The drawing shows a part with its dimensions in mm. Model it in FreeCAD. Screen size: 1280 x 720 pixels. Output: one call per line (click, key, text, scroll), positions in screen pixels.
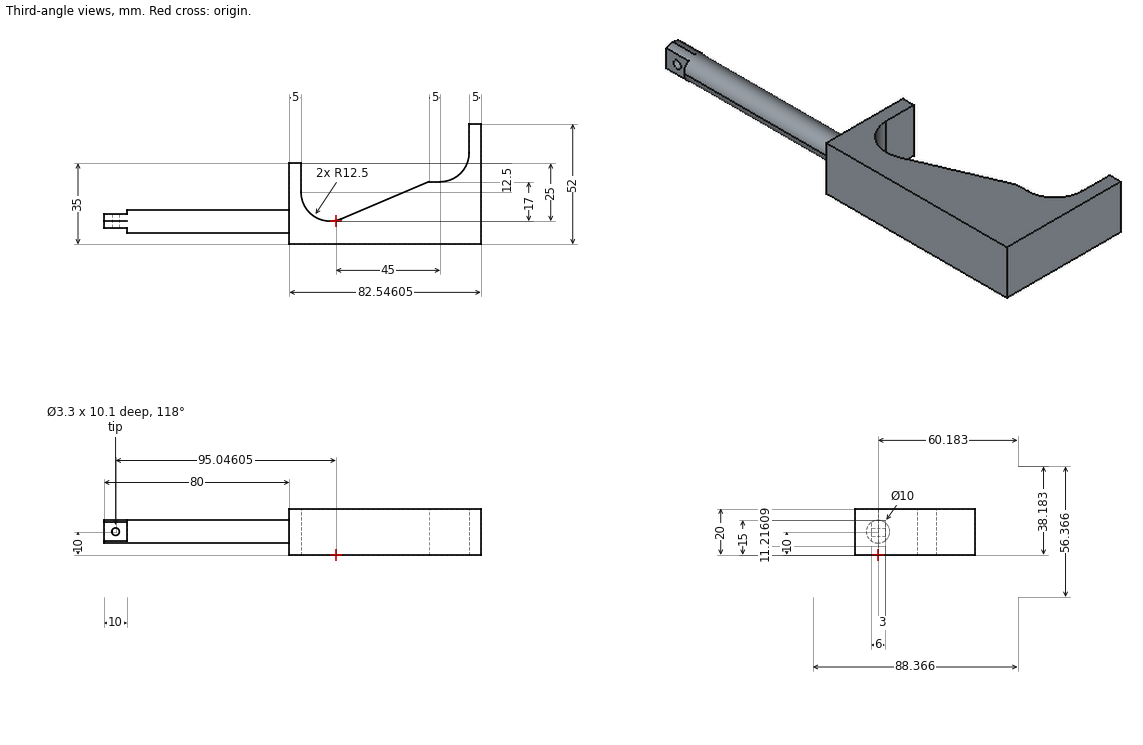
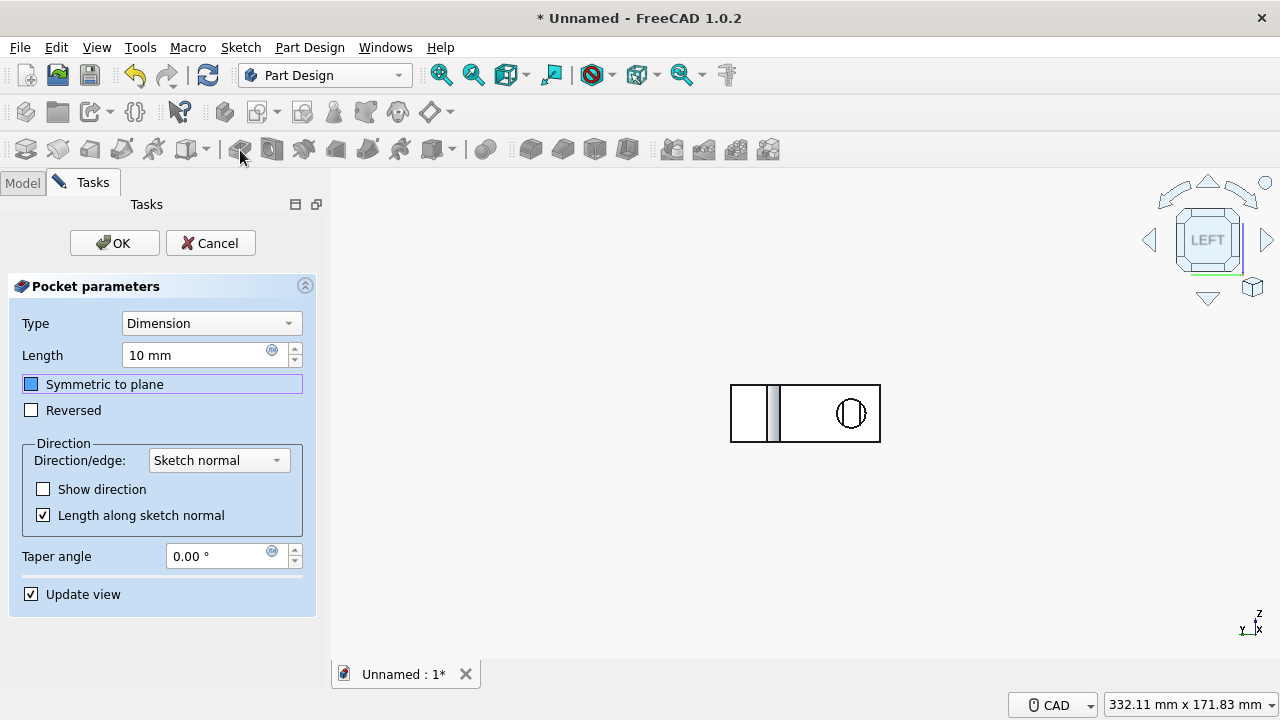
click(115, 243)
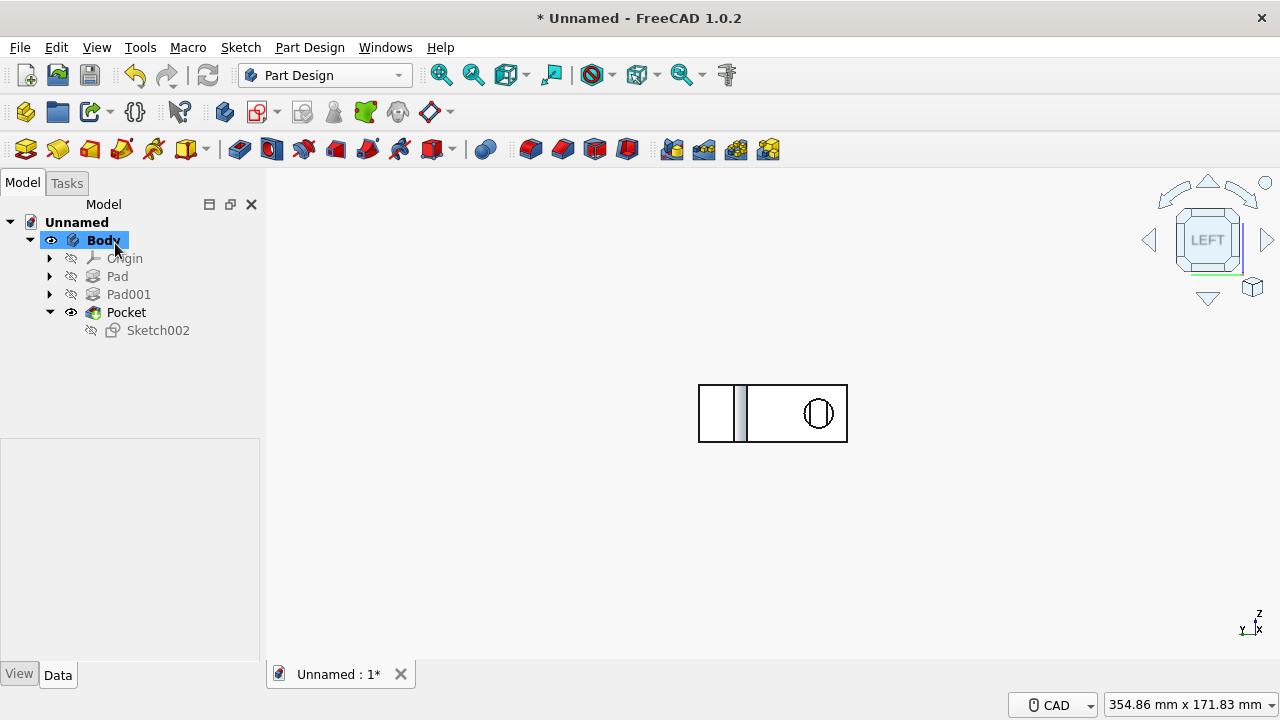
click(442, 76)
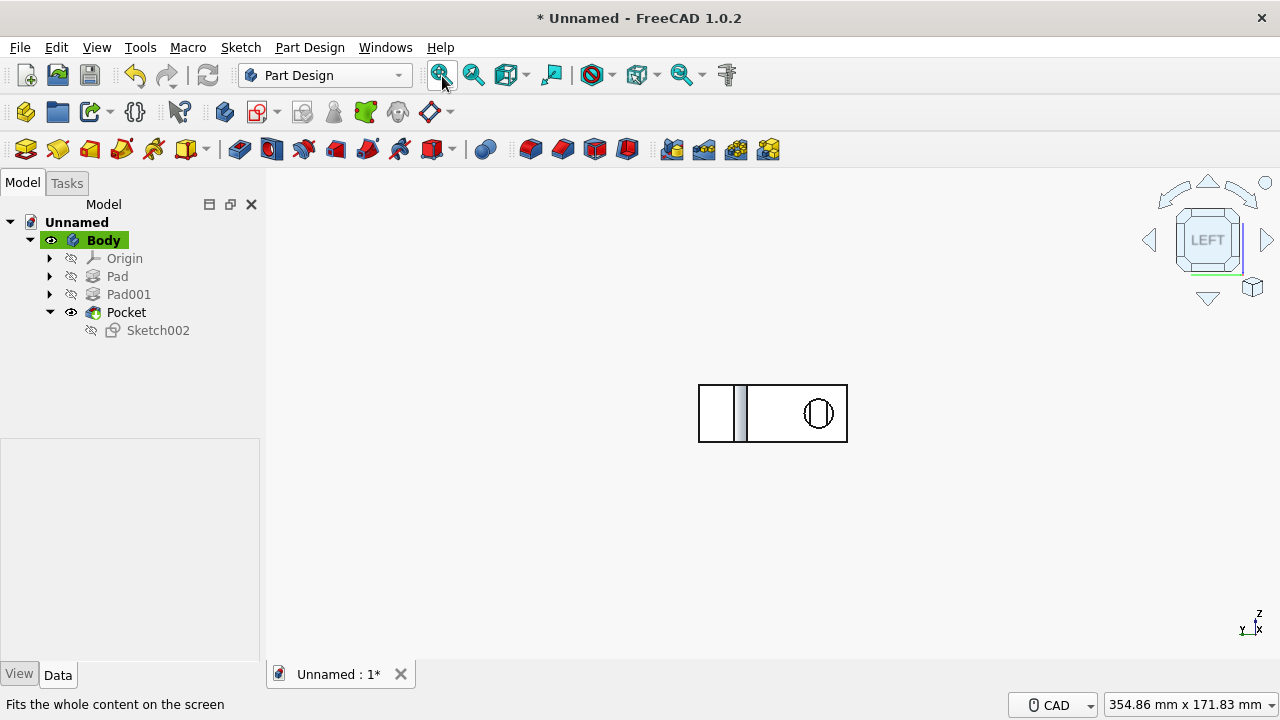
key(4)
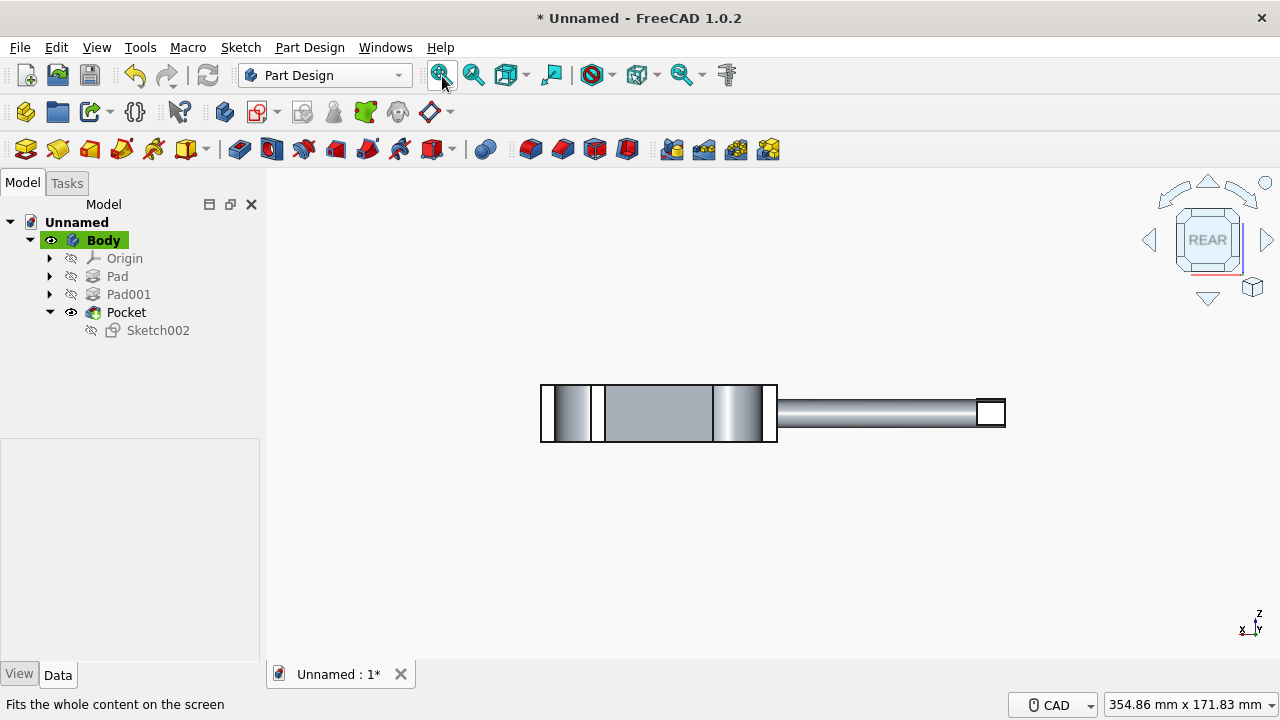
click(991, 412)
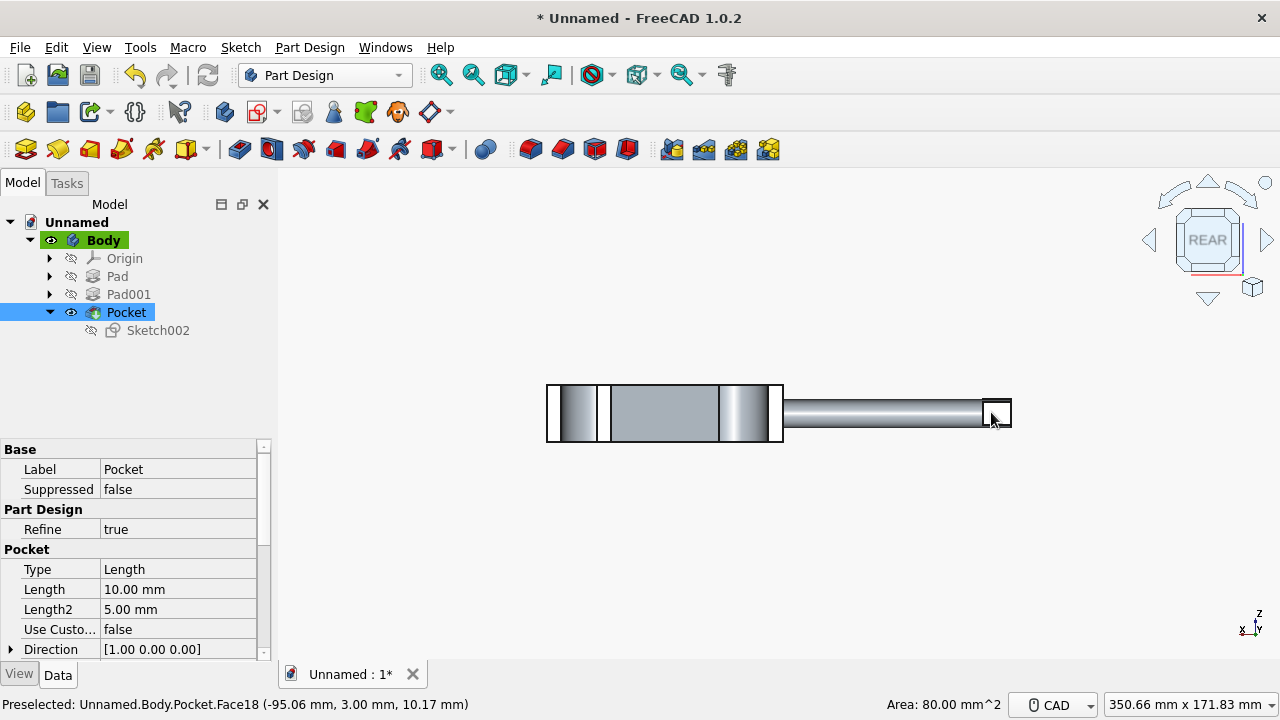
click(258, 112)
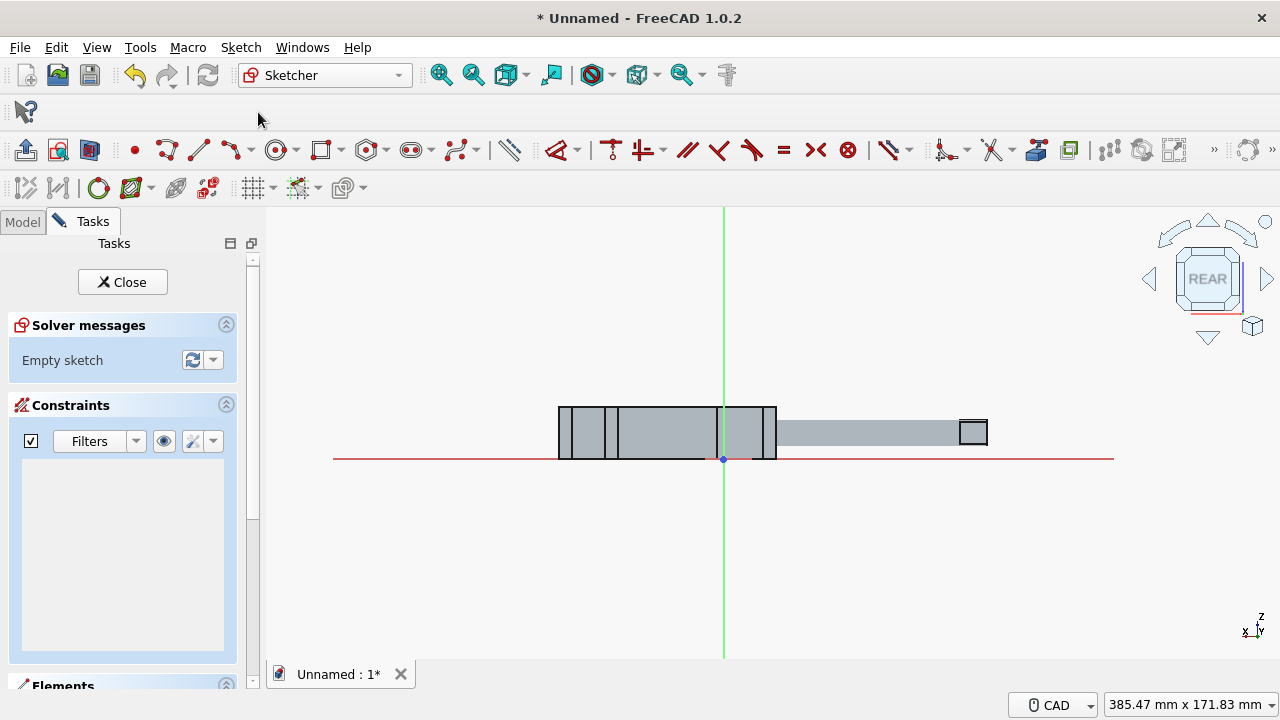
click(90, 150)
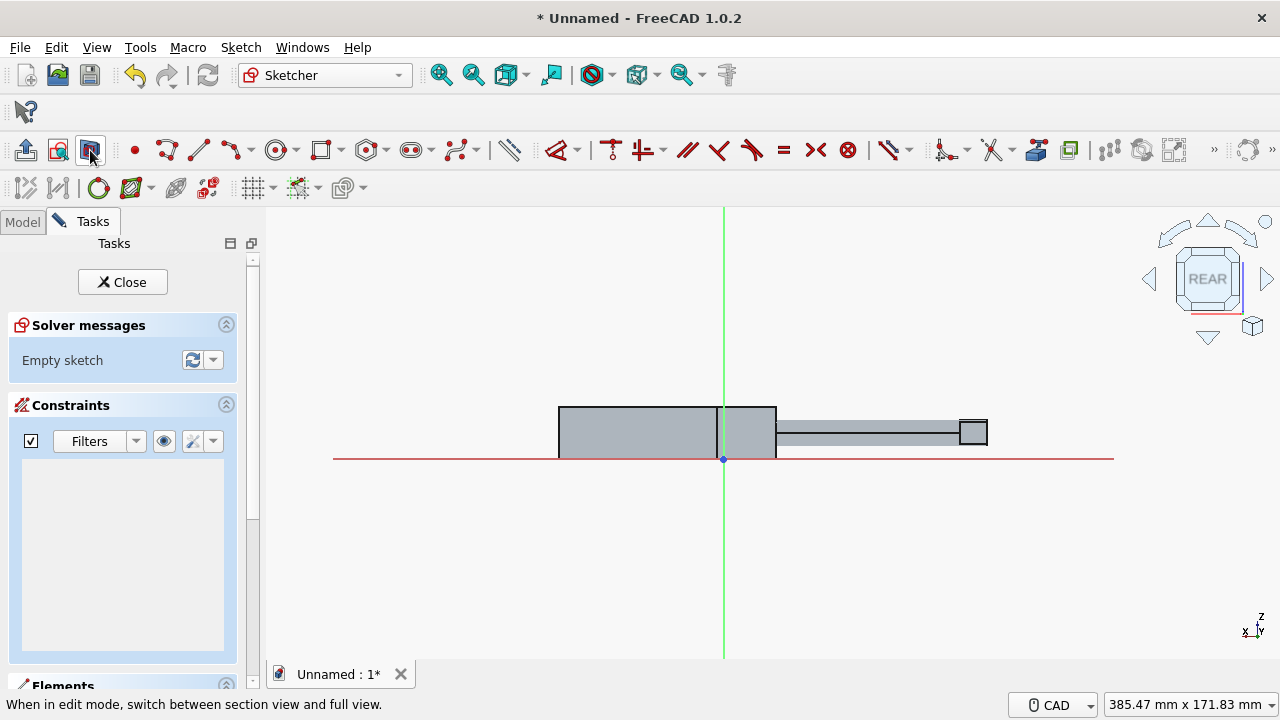
scroll(988, 433, up, 15)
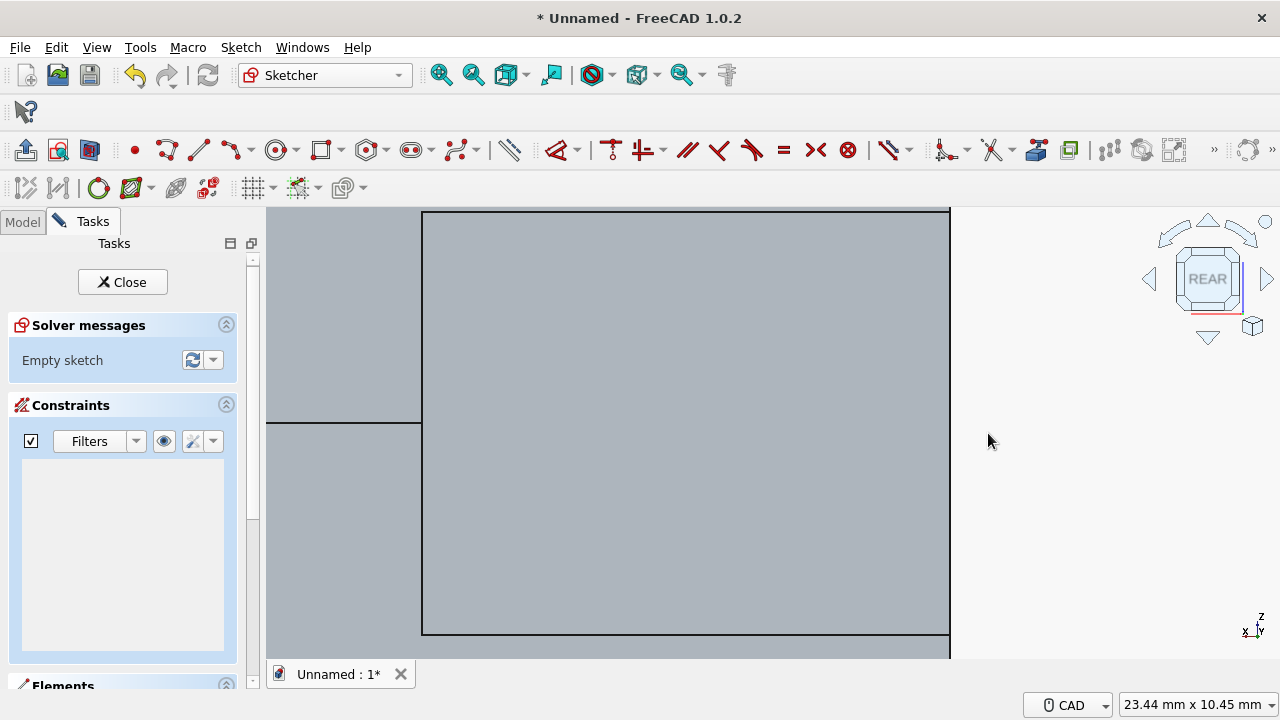
scroll(648, 404, up, 2)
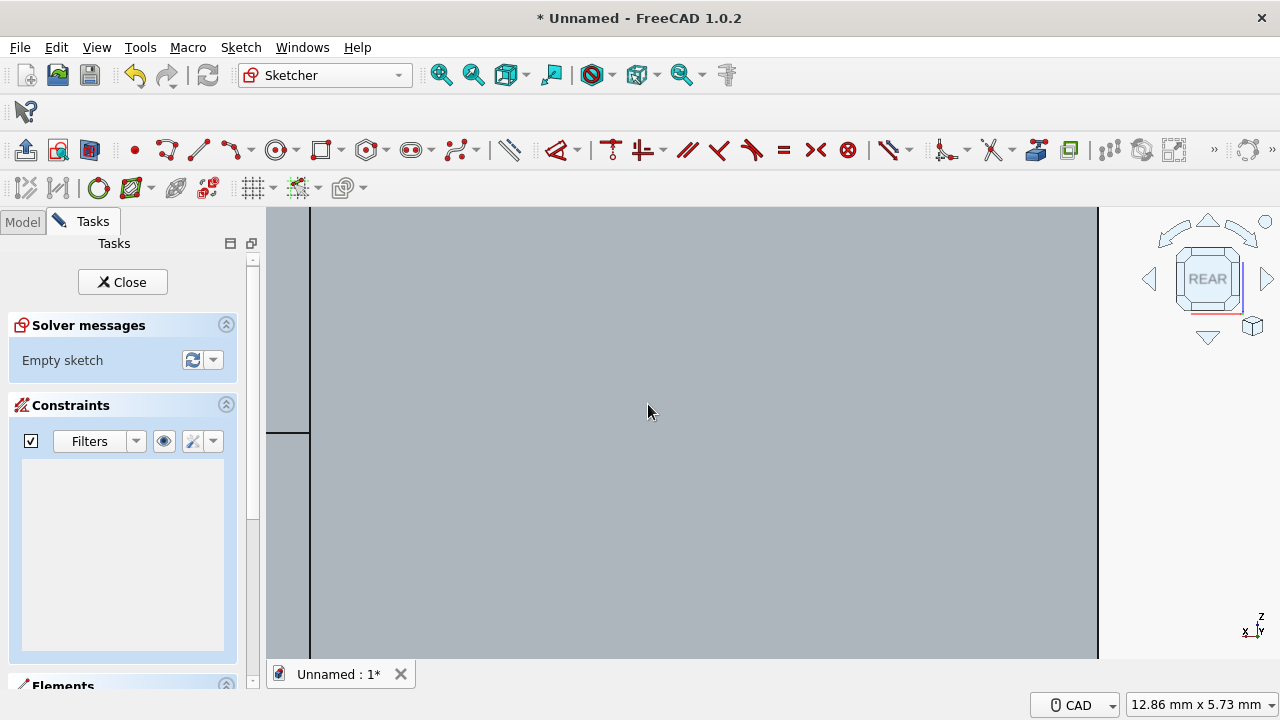
click(276, 150)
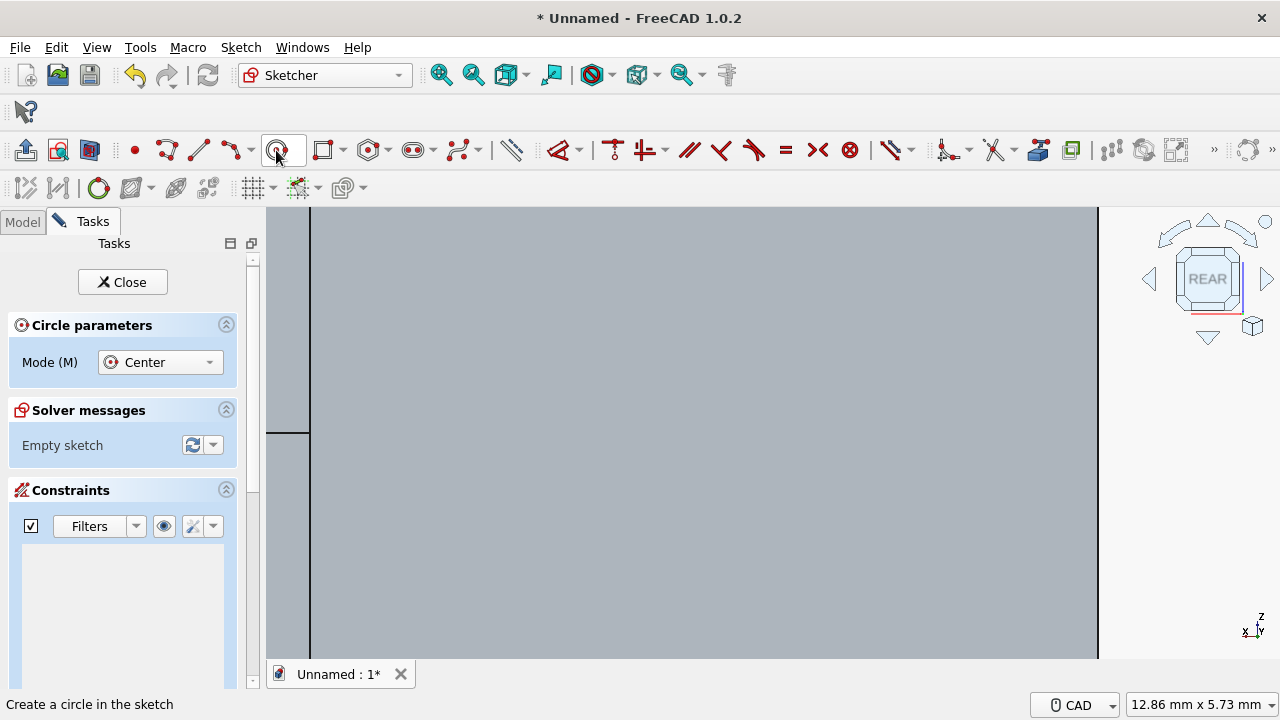
click(704, 433)
click(796, 341)
key(Escape)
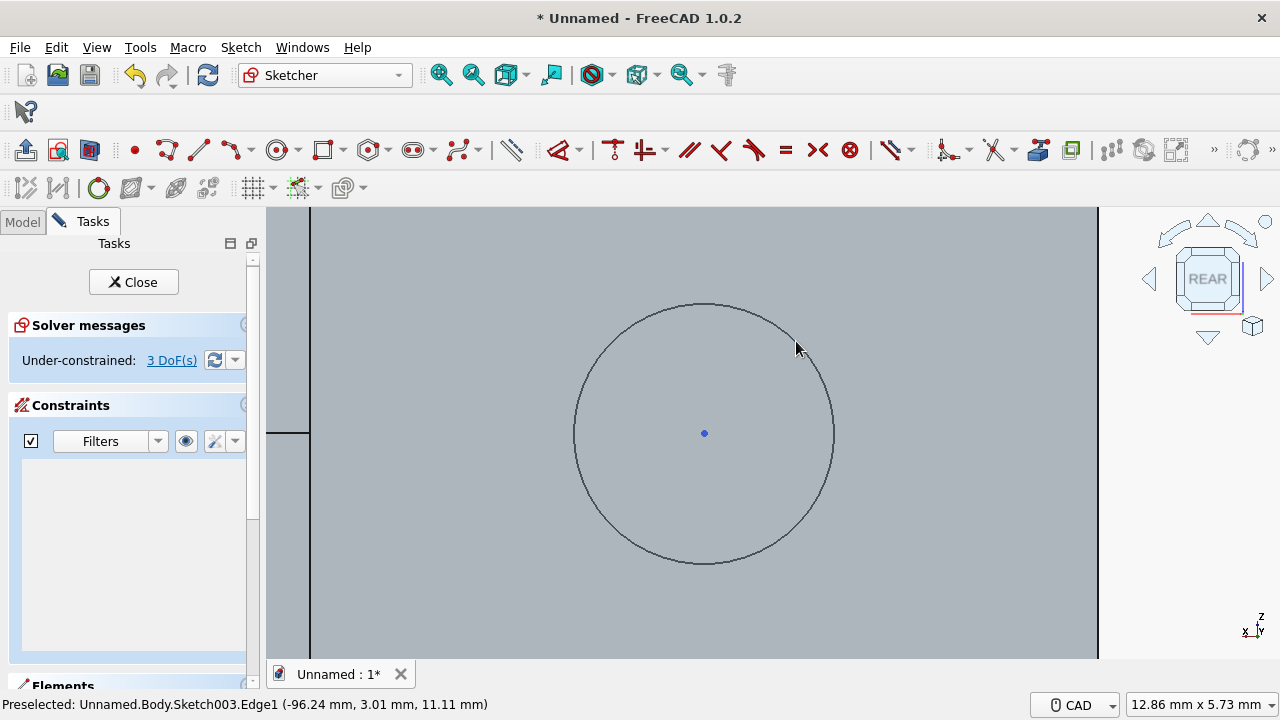
click(558, 150)